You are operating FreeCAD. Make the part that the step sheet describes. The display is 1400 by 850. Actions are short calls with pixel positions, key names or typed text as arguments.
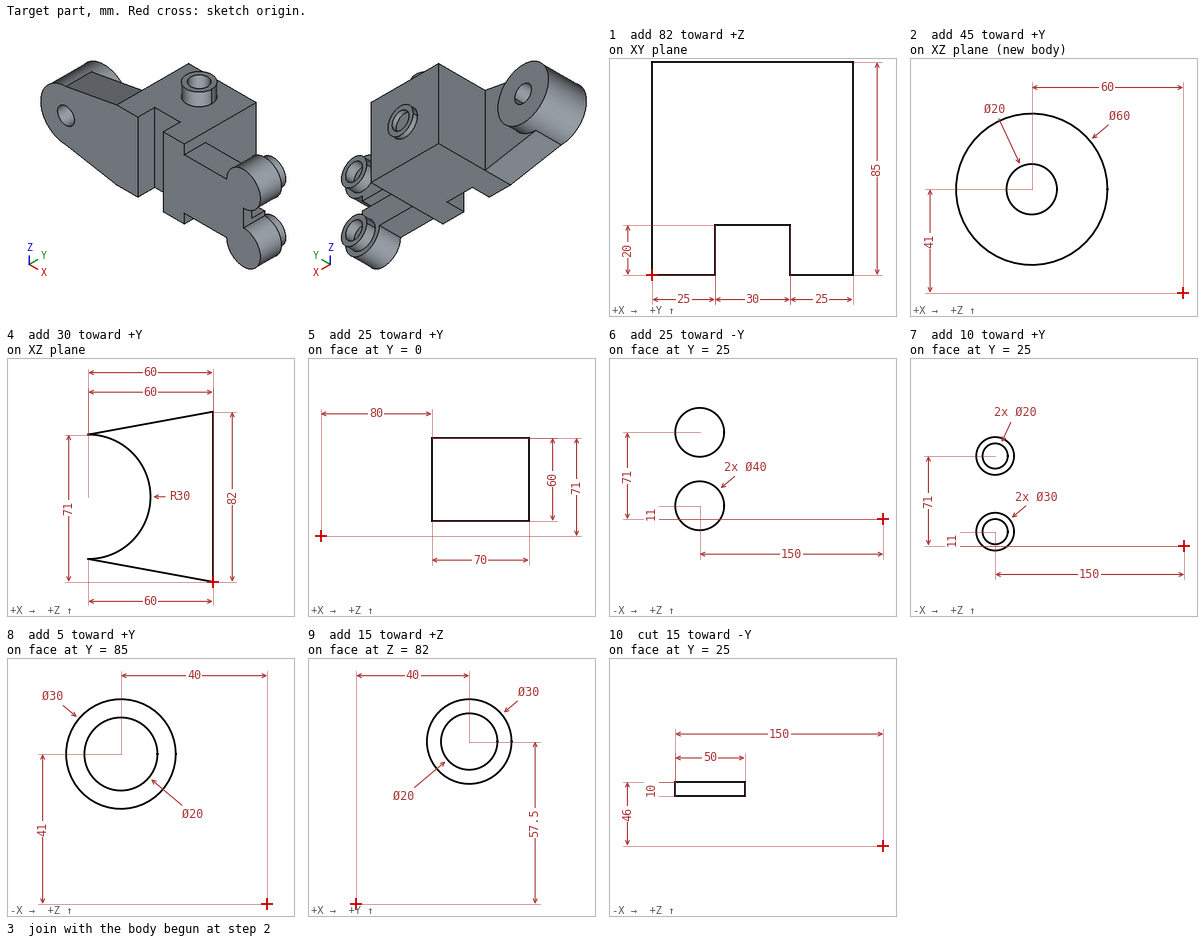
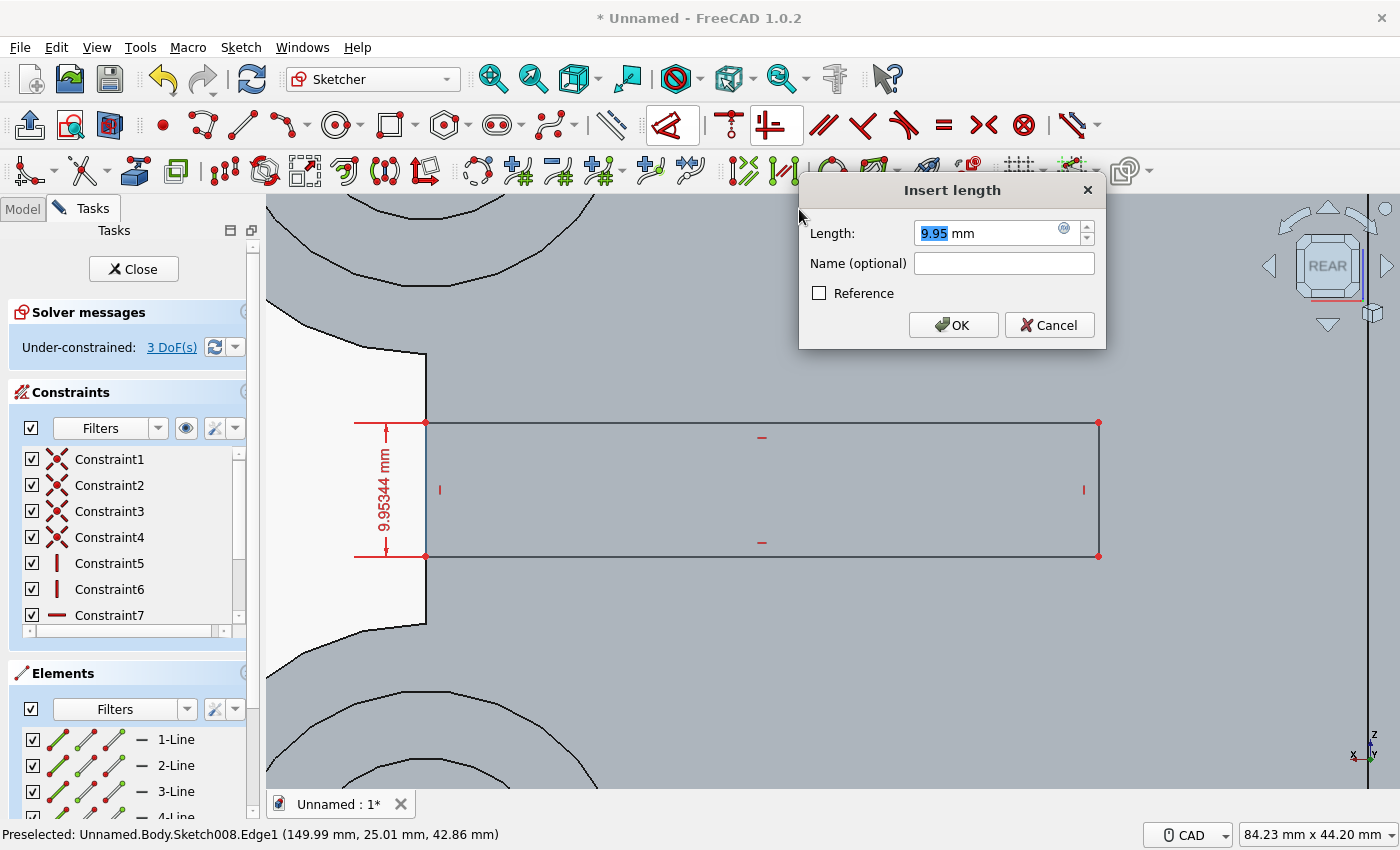
text(10)
key(Return)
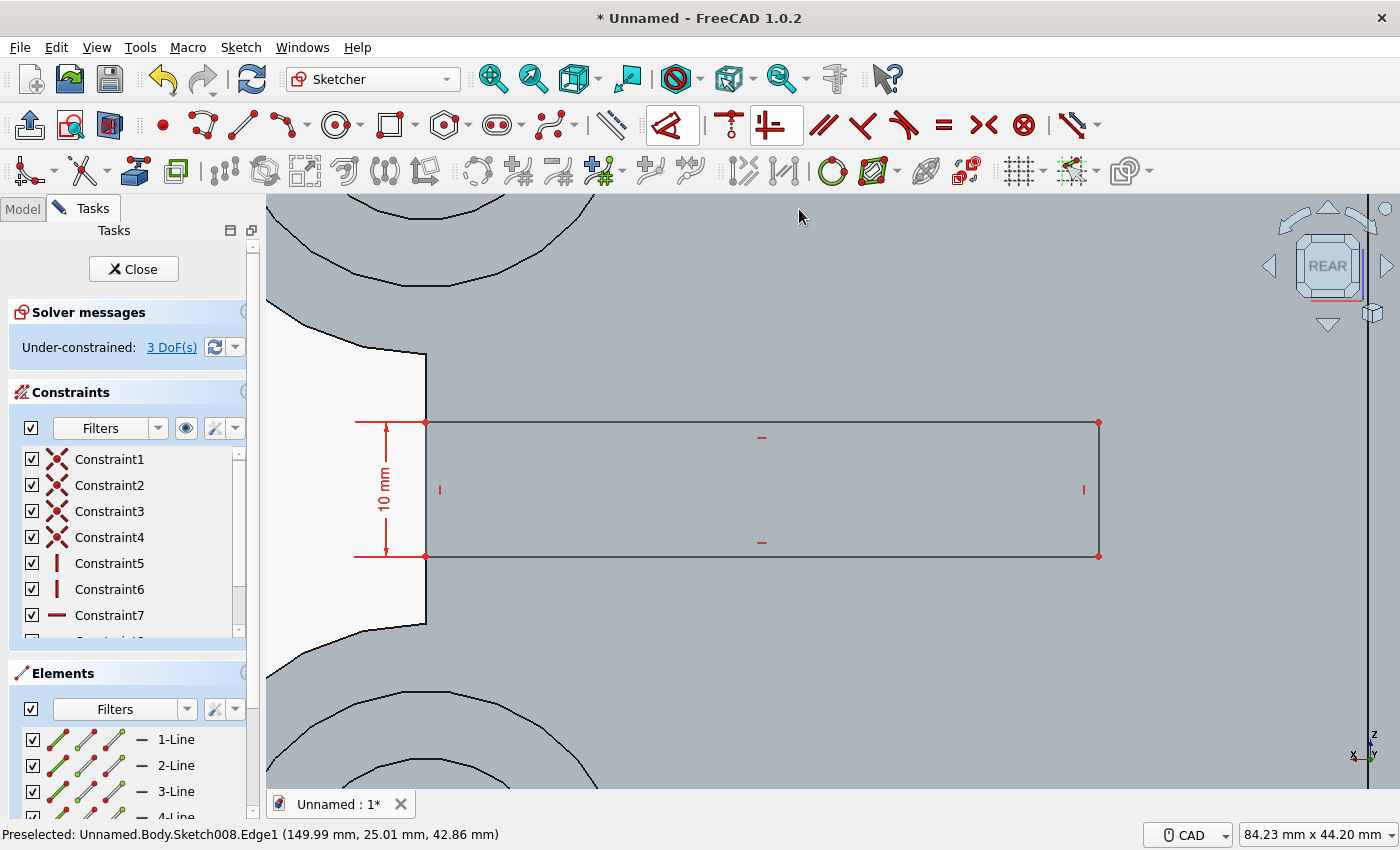
click(628, 557)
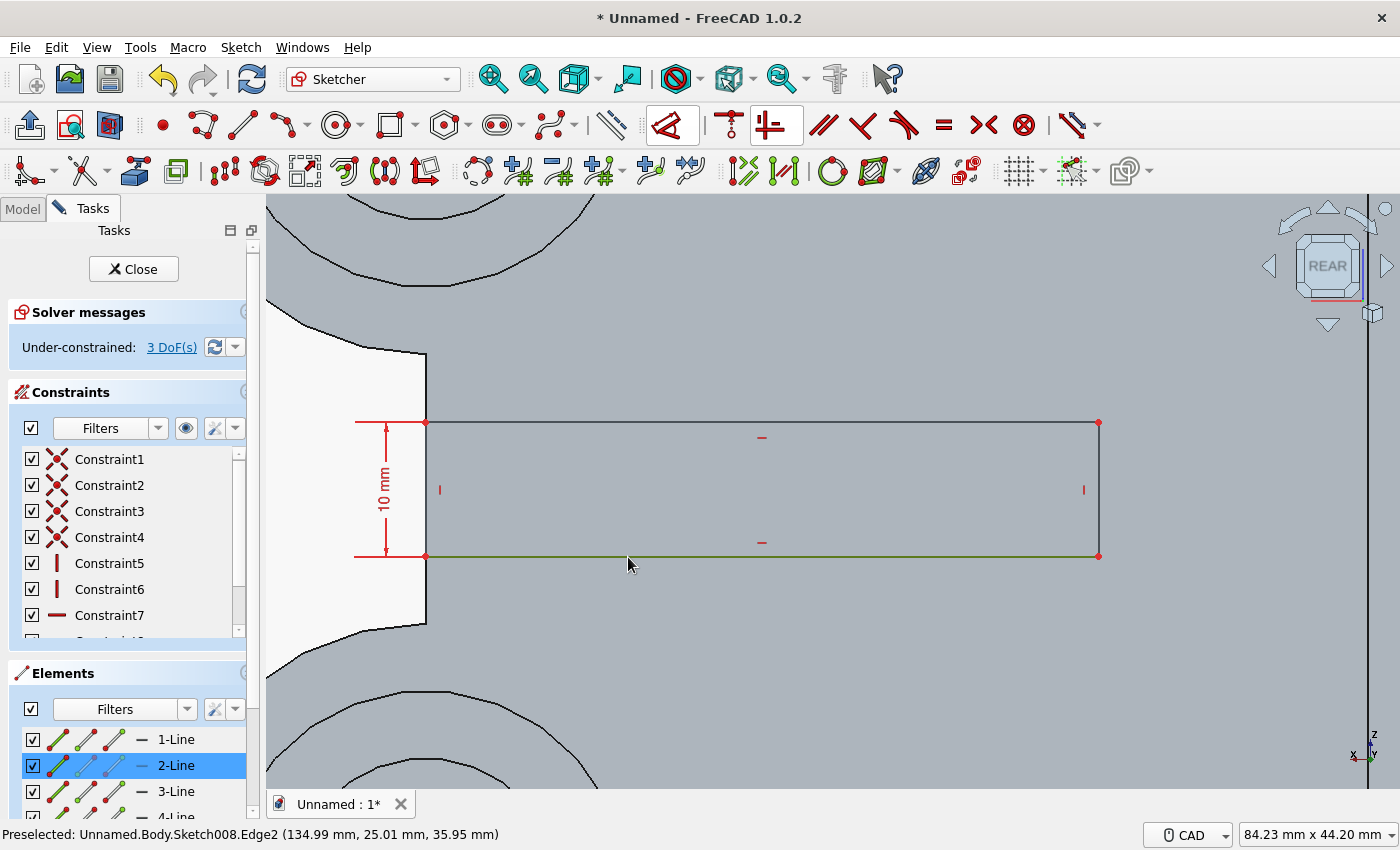
click(694, 126)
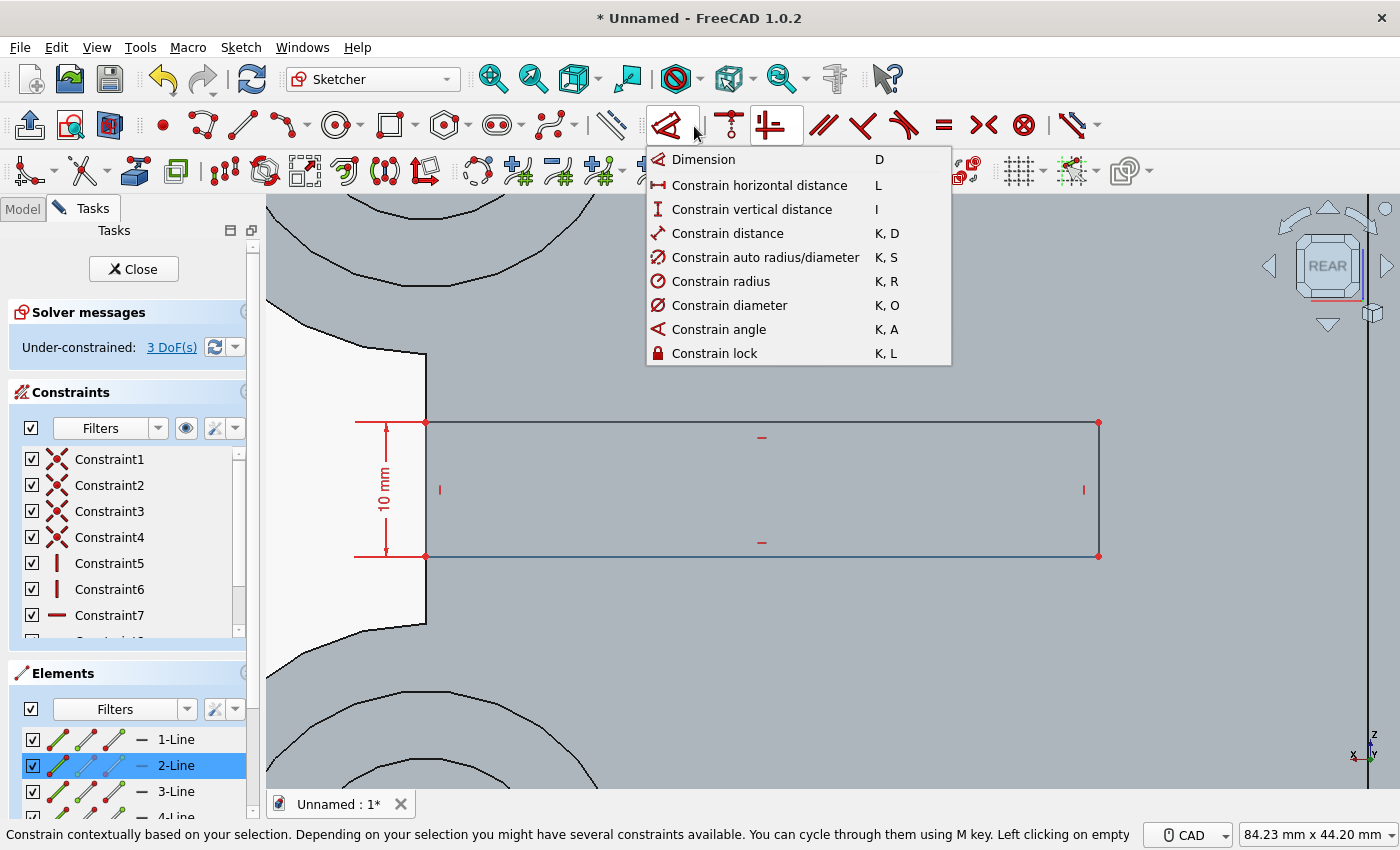
click(799, 185)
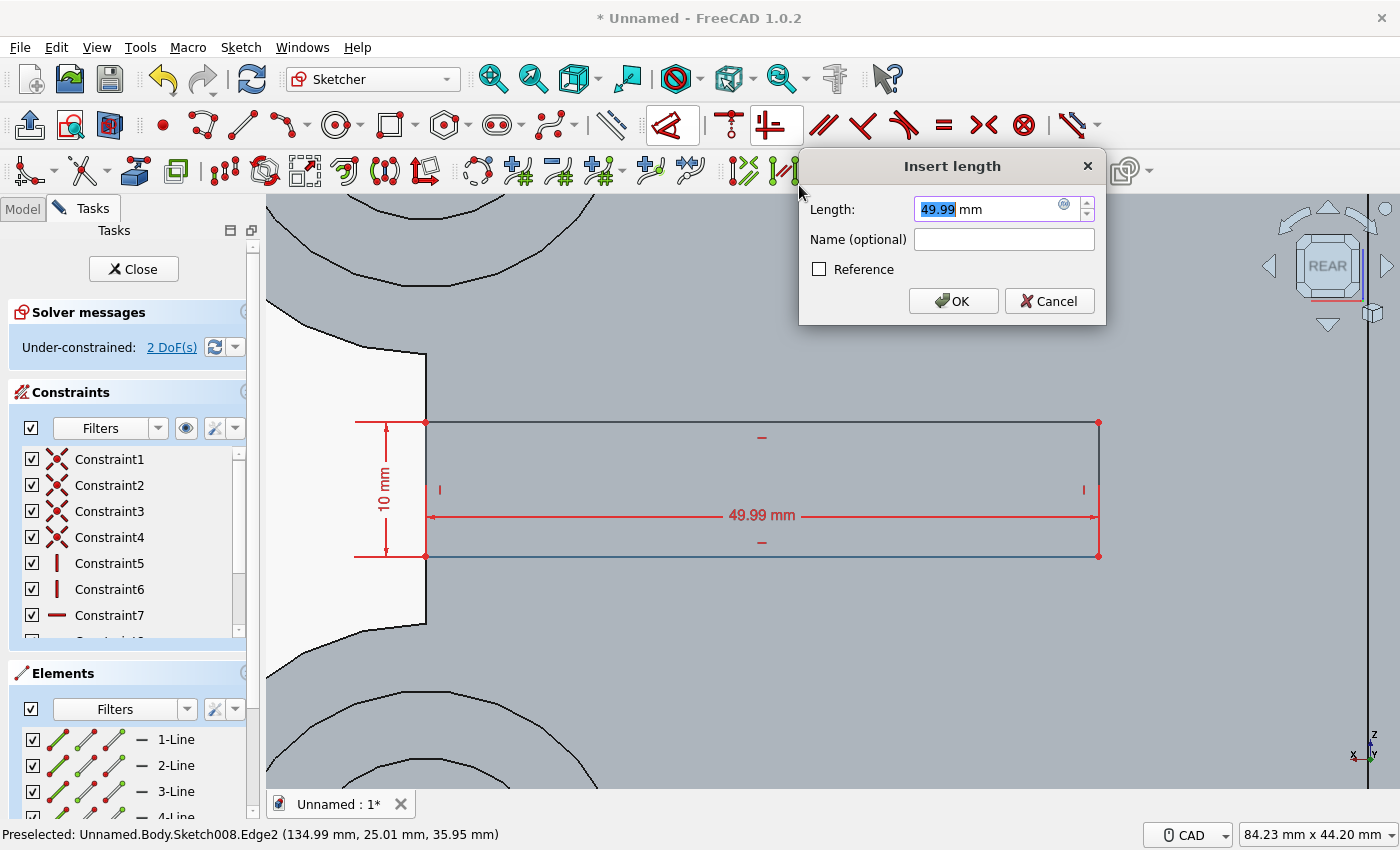
text(50)
key(Return)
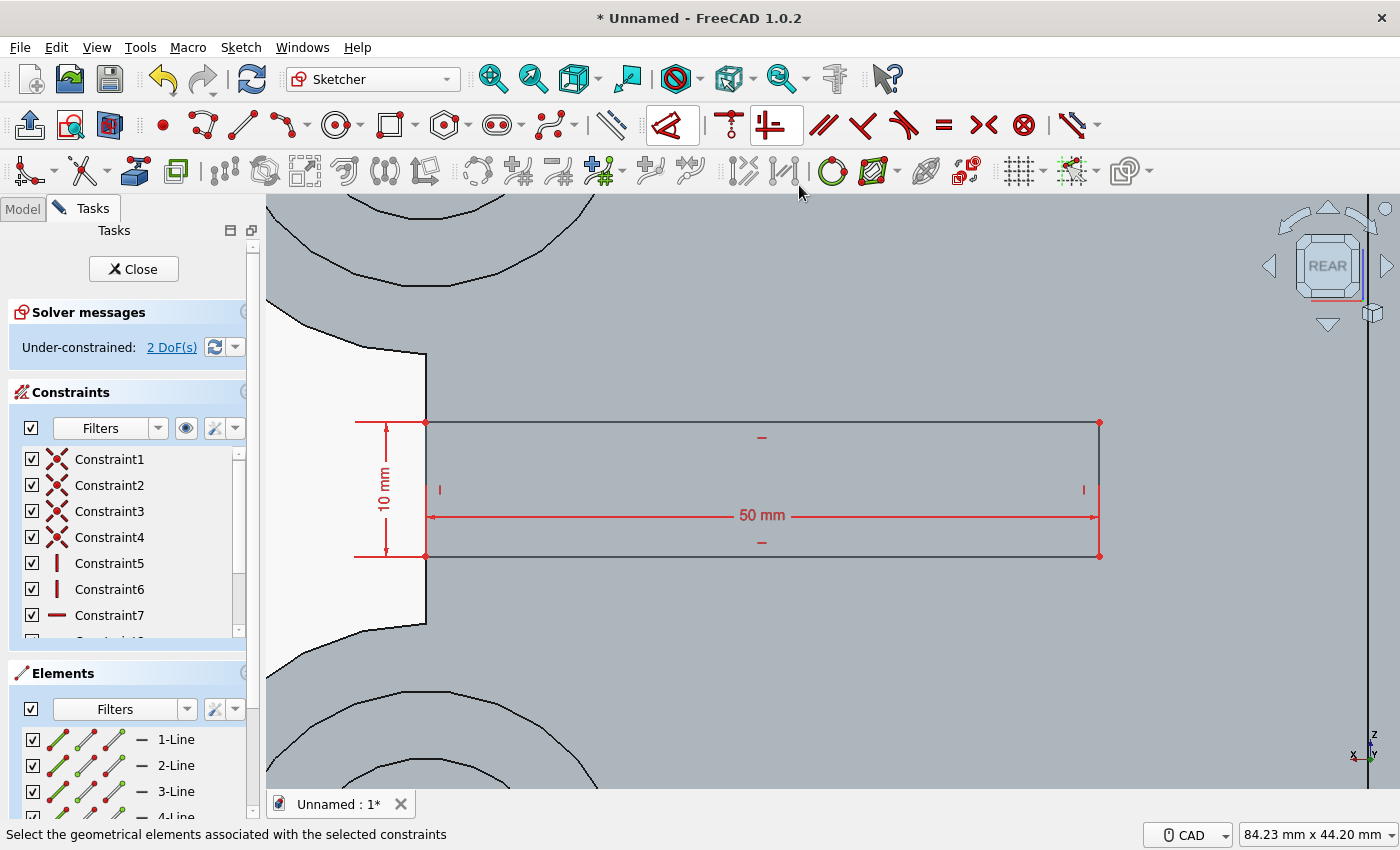
click(426, 422)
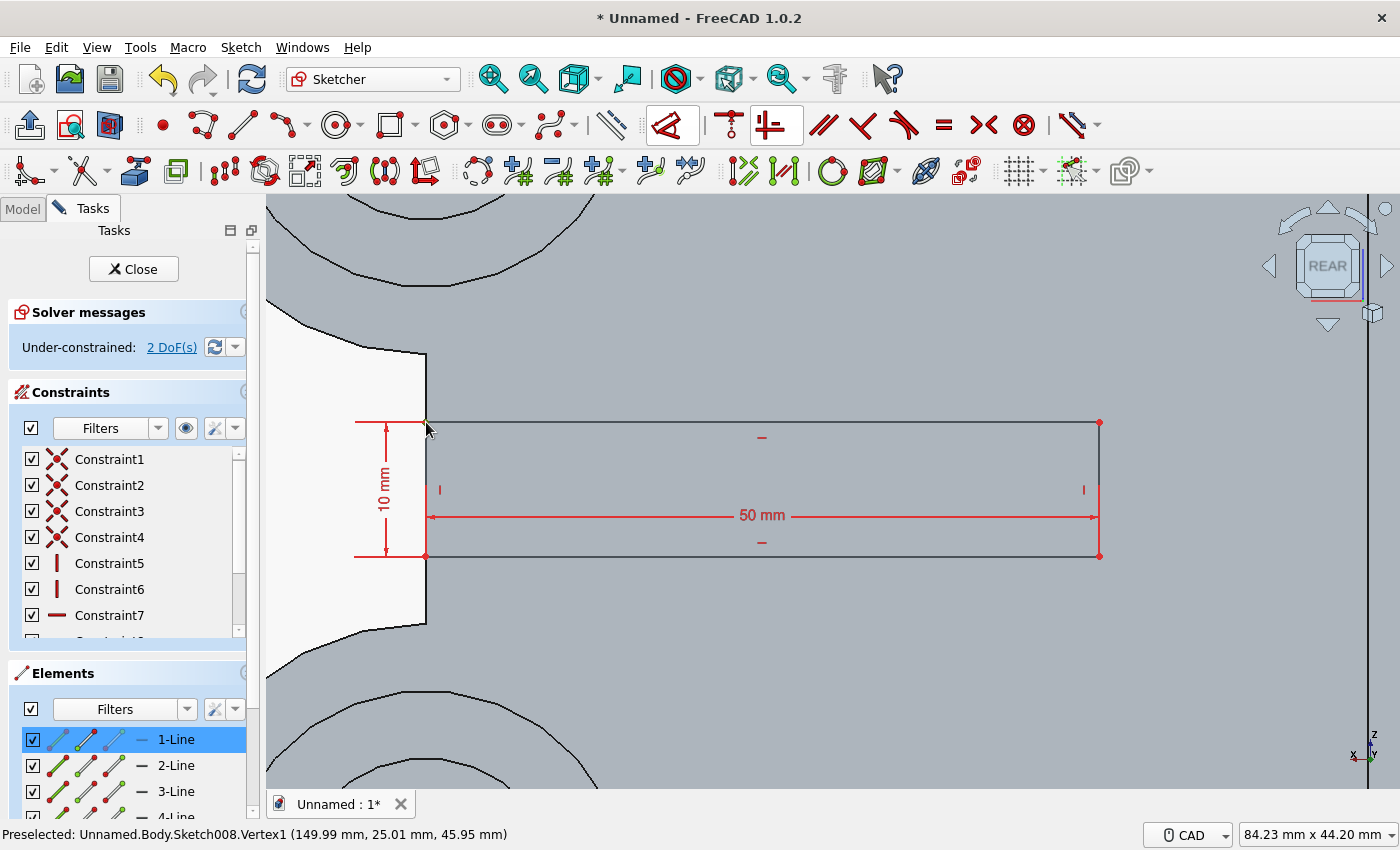
key(i)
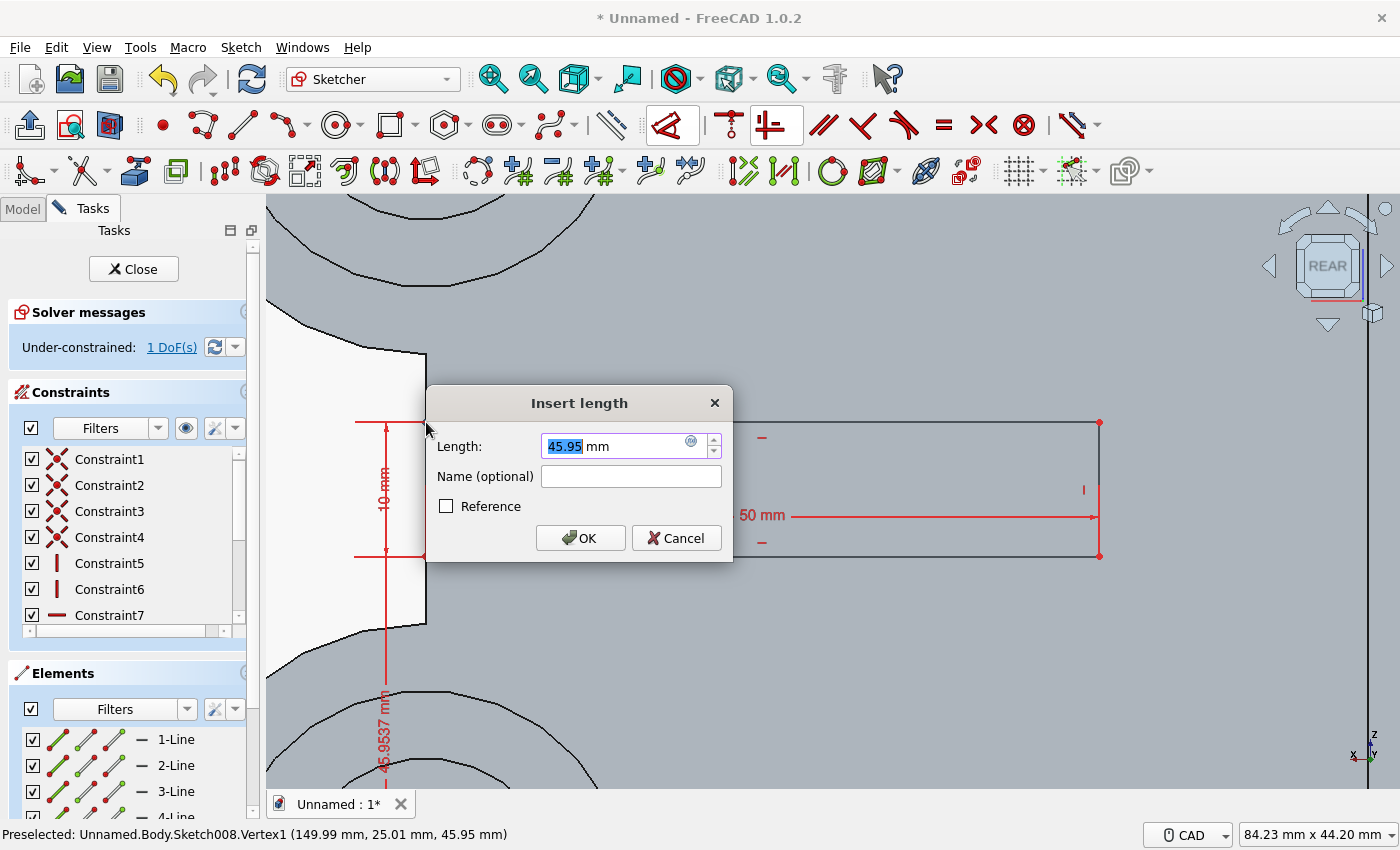
text(46)
key(Return)